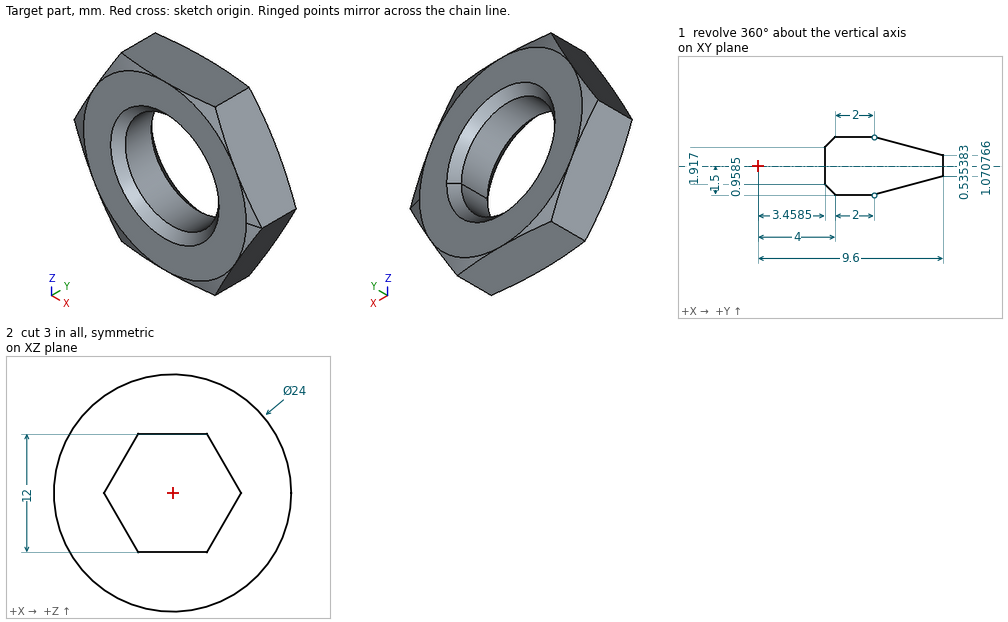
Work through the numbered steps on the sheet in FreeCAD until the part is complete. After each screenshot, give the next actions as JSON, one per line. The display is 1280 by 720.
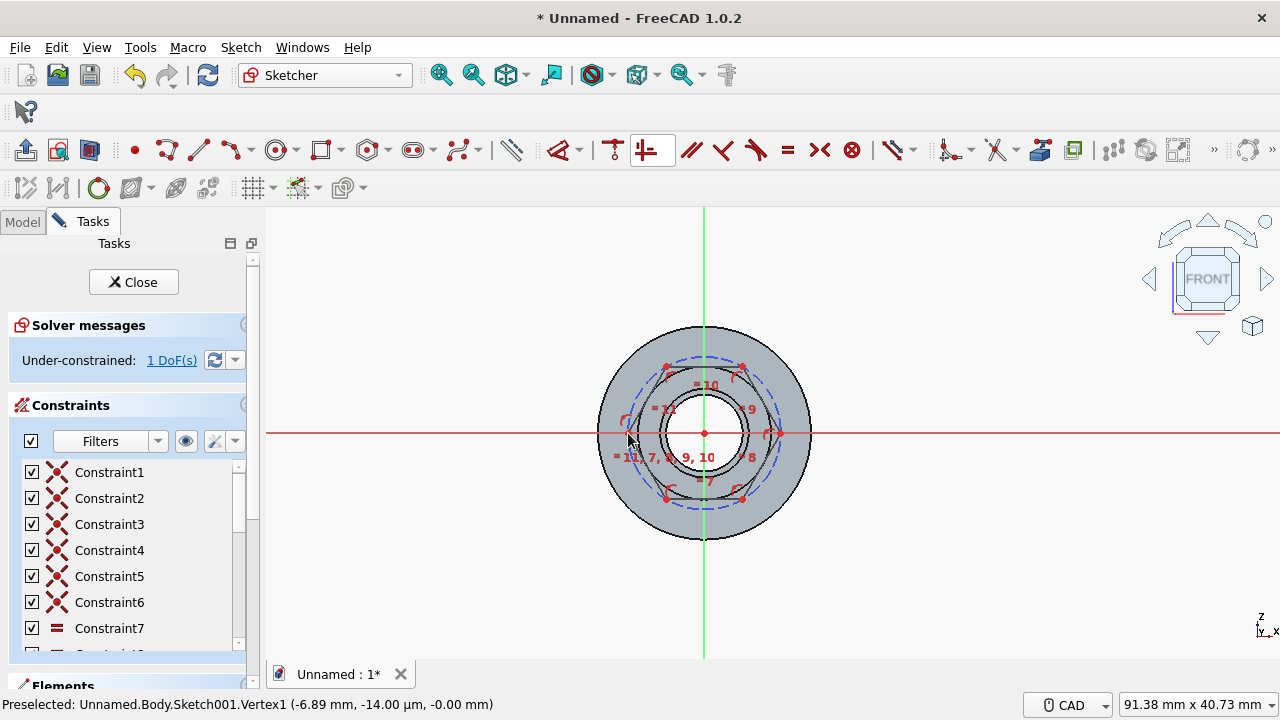
{"action": "left_click", "coordinate": [276, 150]}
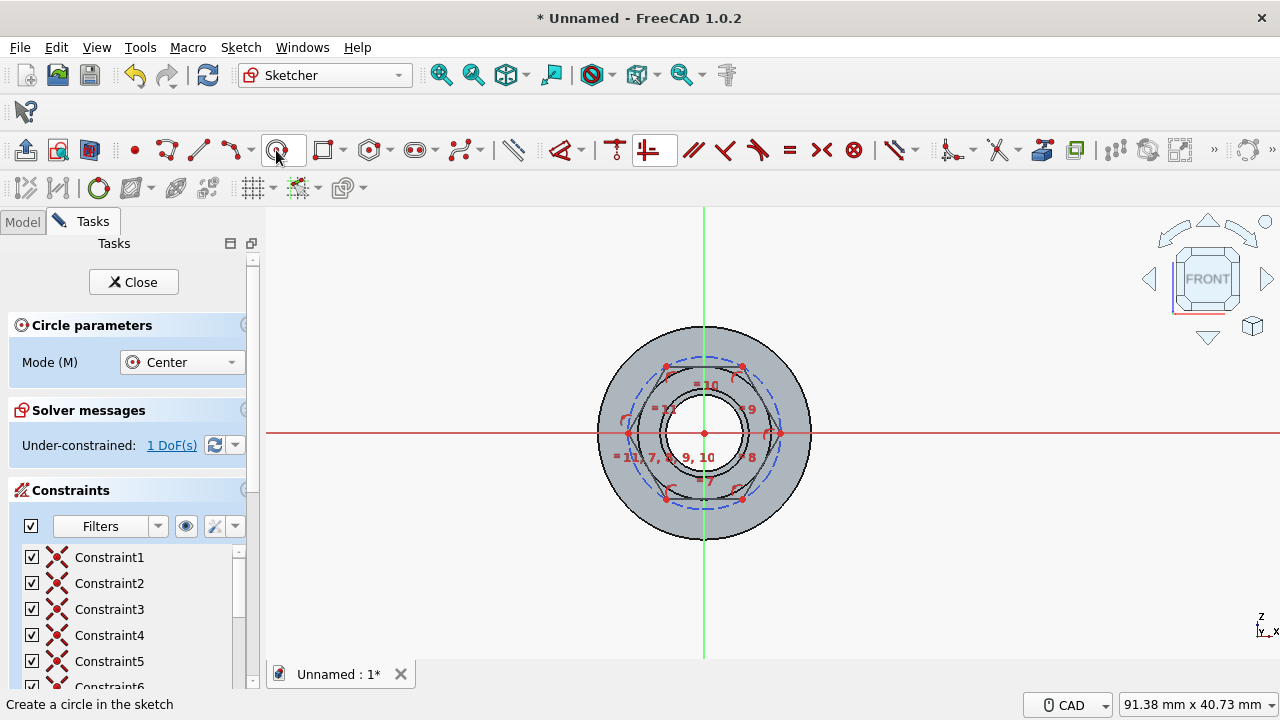
{"action": "left_click", "coordinate": [704, 433]}
{"action": "left_click", "coordinate": [799, 339]}
{"action": "key", "text": "Escape"}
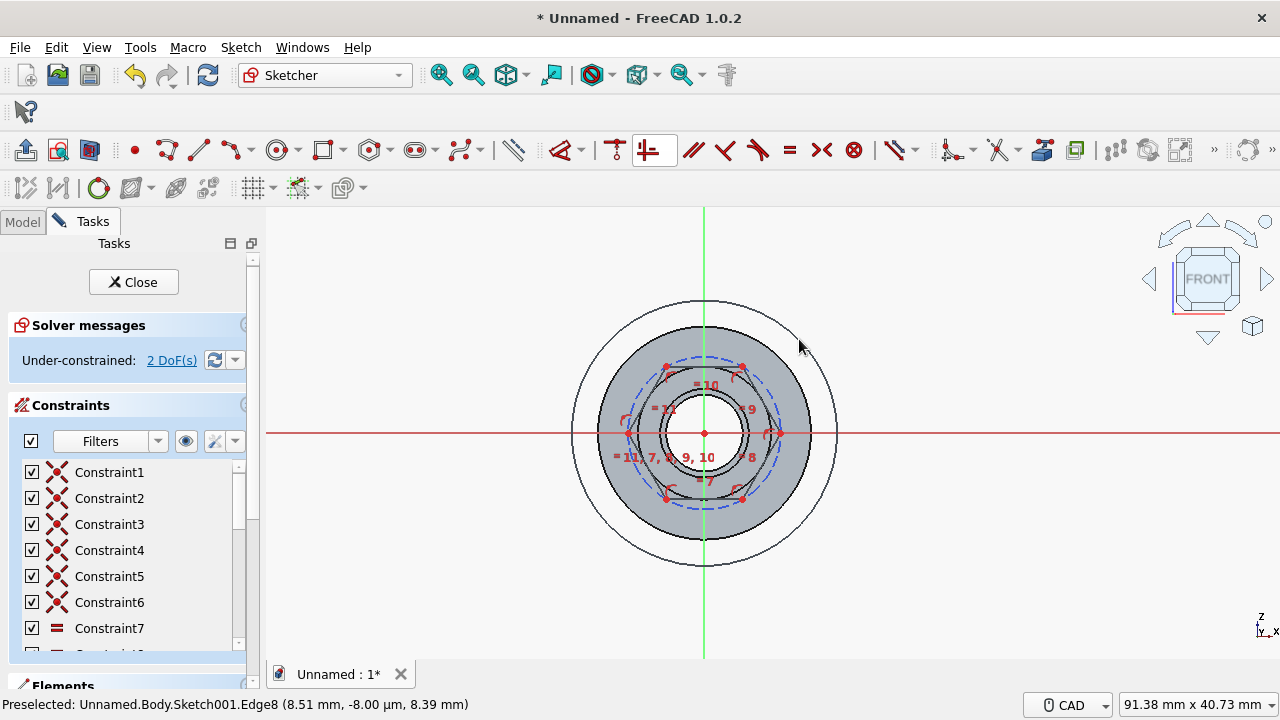
{"action": "left_click", "coordinate": [560, 150]}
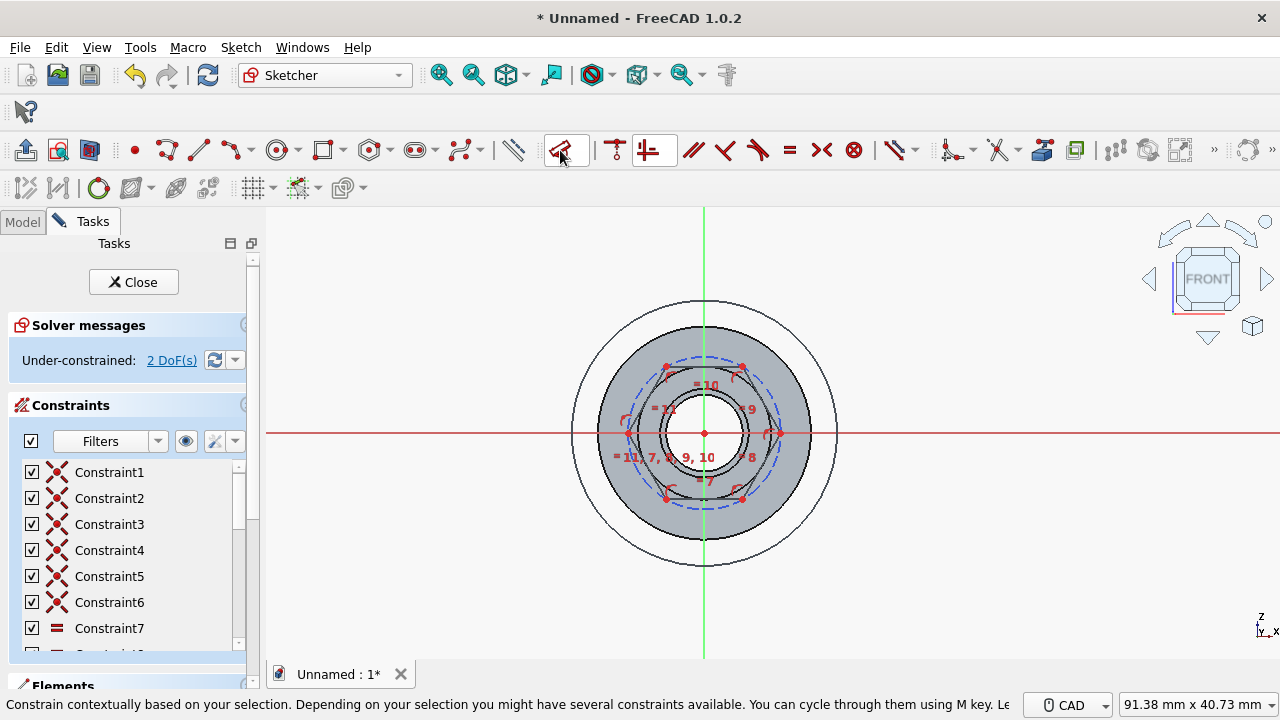
{"action": "left_click", "coordinate": [798, 339]}
{"action": "left_click", "coordinate": [821, 316]}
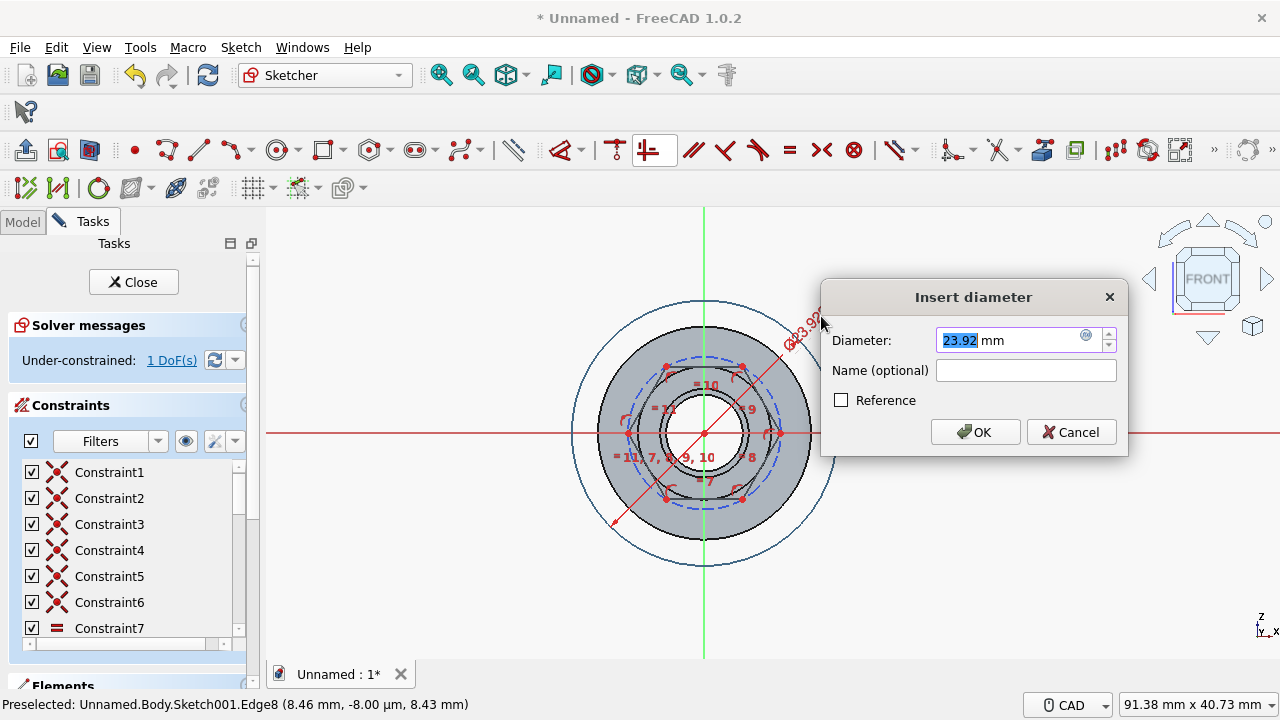
{"action": "type", "text": "24"}
{"action": "key", "text": "Return"}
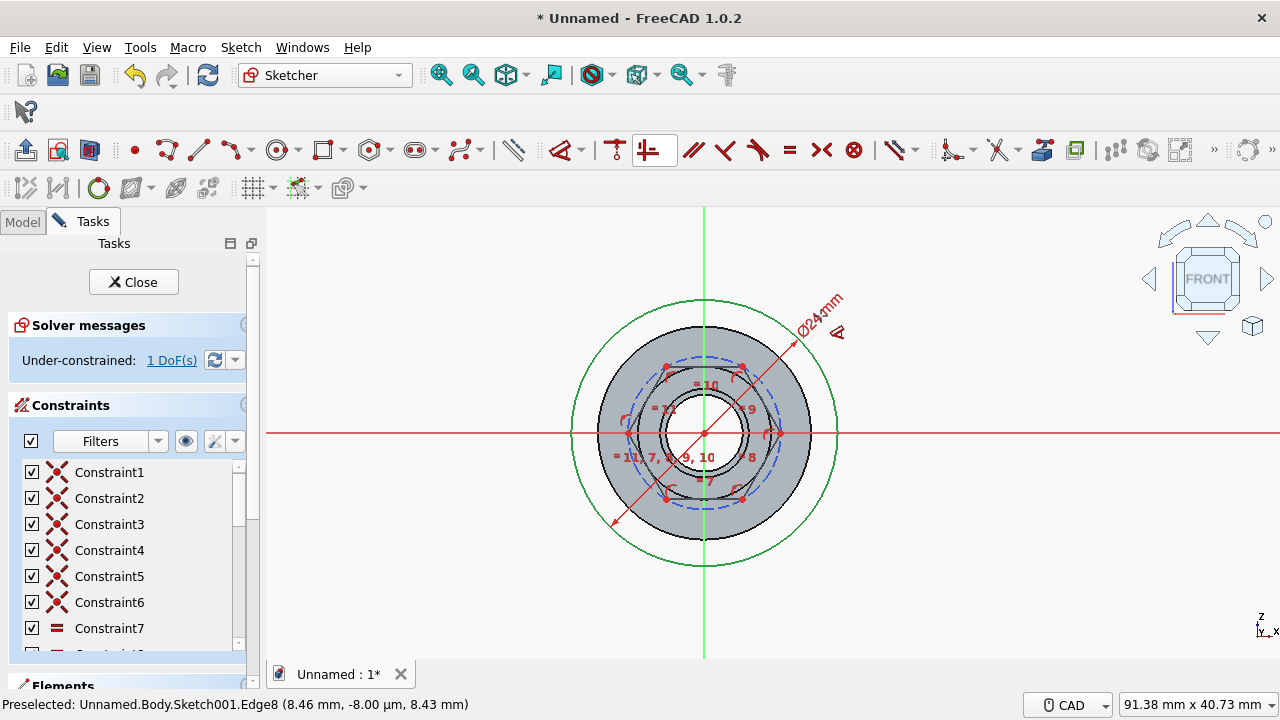
{"action": "left_click", "coordinate": [666, 499]}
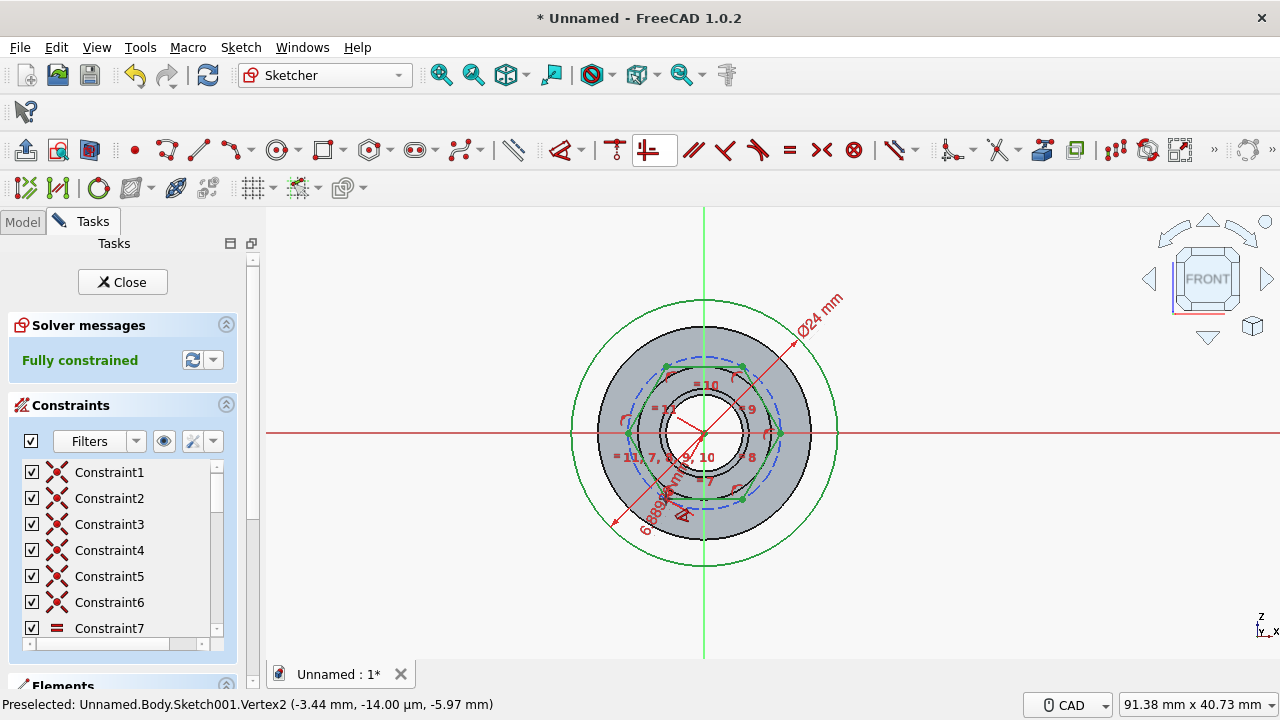
{"action": "left_click", "coordinate": [743, 367]}
{"action": "left_click", "coordinate": [801, 403]}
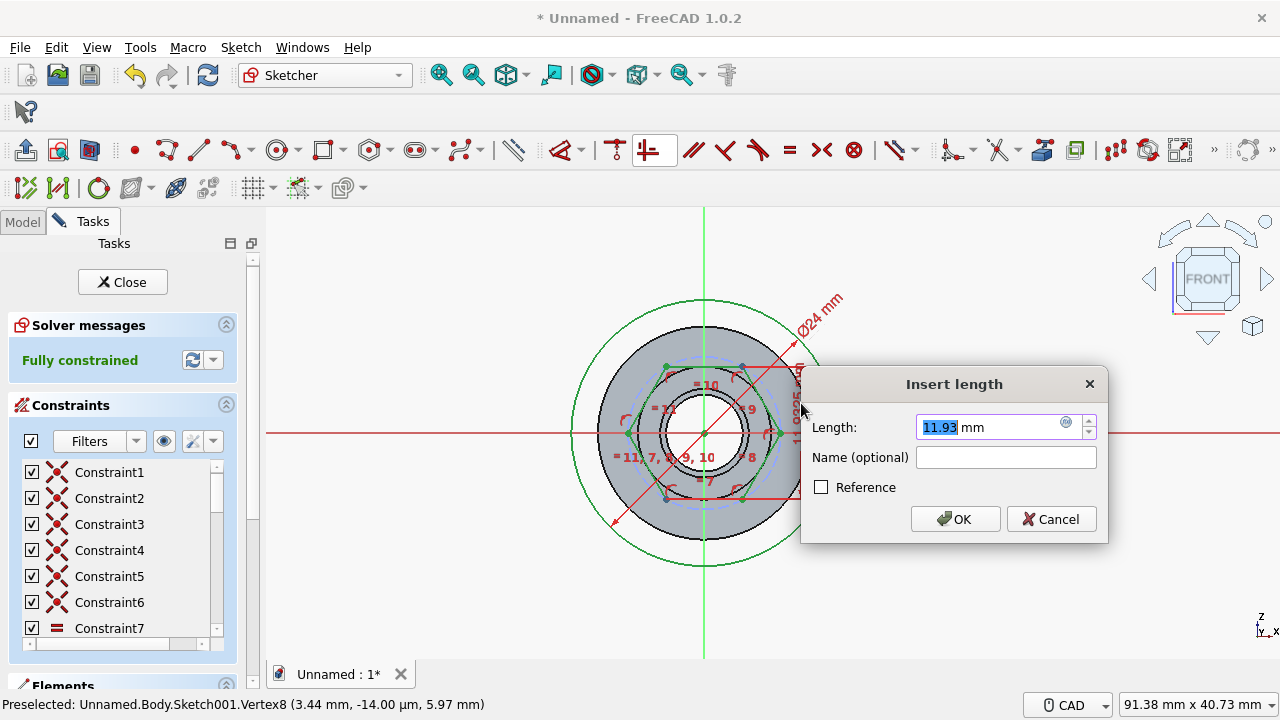
{"action": "type", "text": "12"}
{"action": "key", "text": "Return"}
{"action": "key", "text": "Escape"}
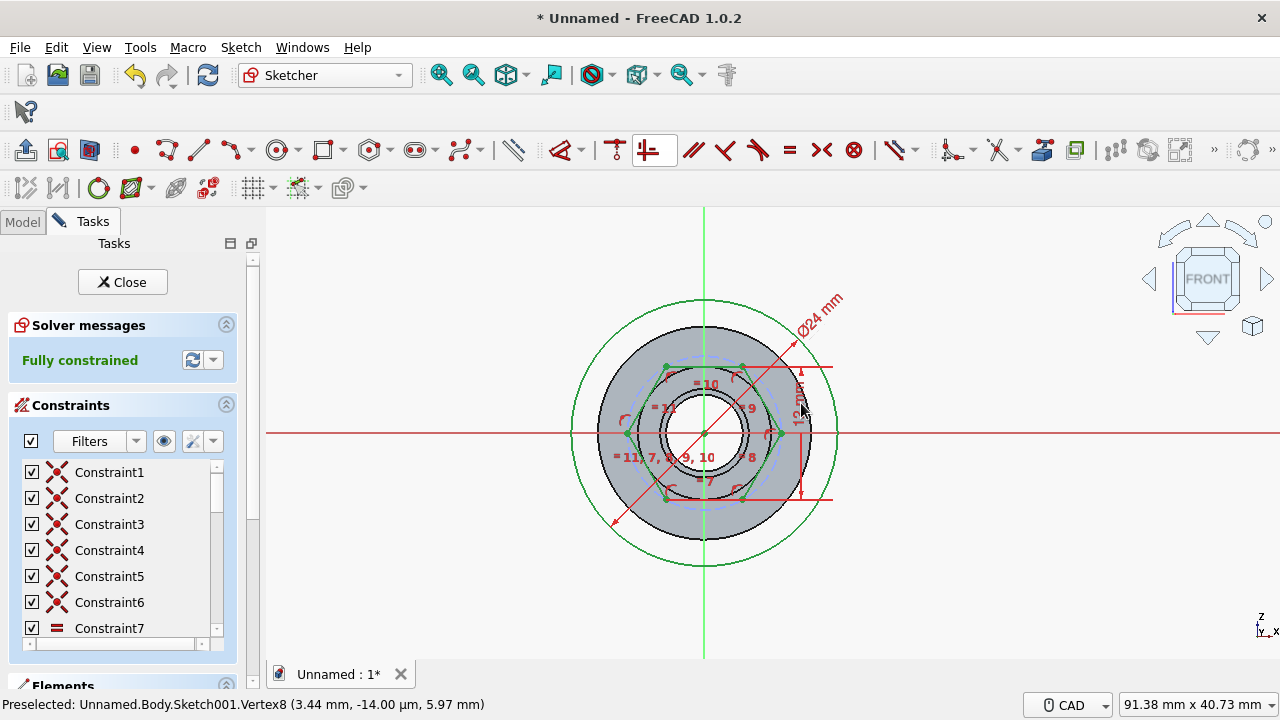
{"action": "left_click", "coordinate": [123, 282]}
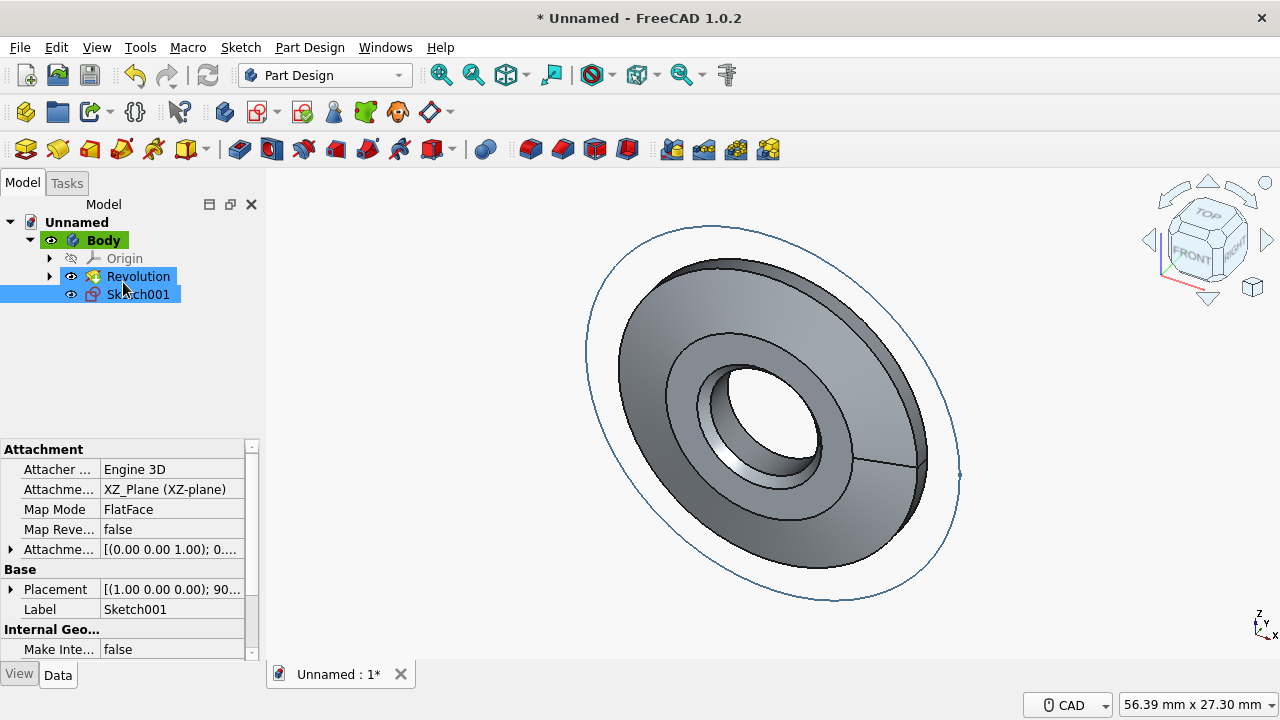
{"action": "left_click", "coordinate": [240, 150]}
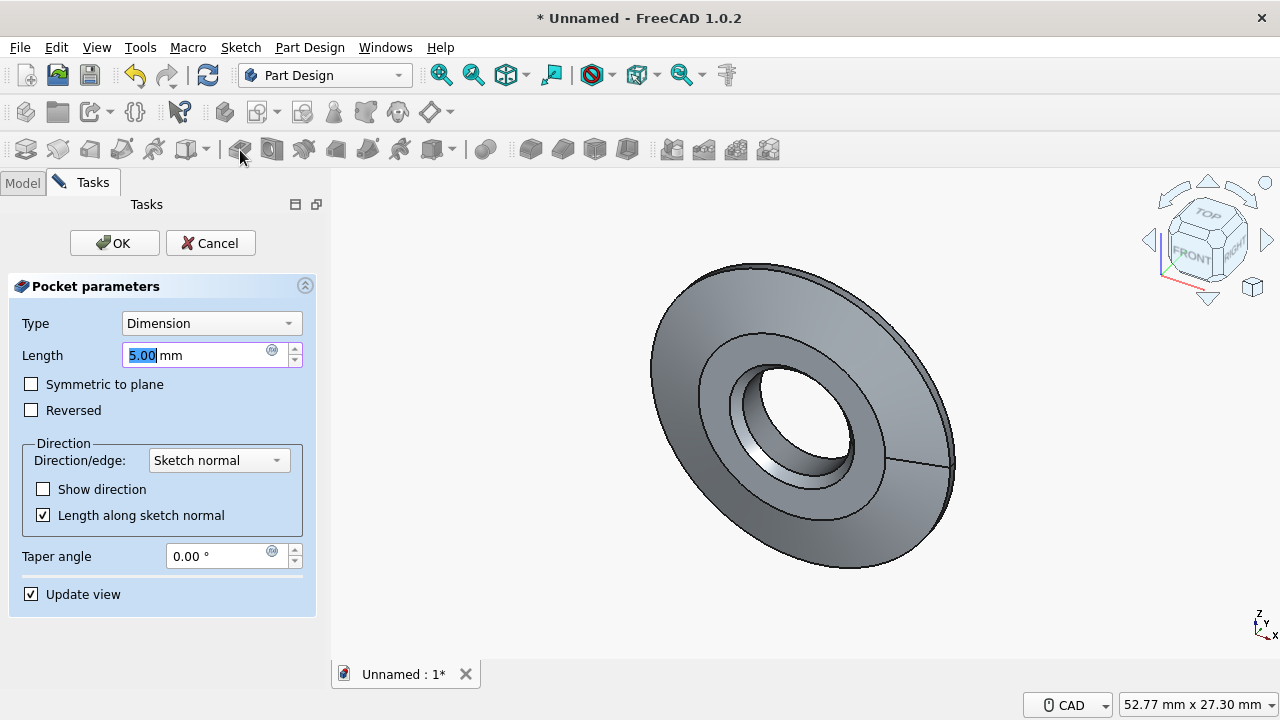
{"action": "type", "text": "3"}
{"action": "key", "text": "Tab"}